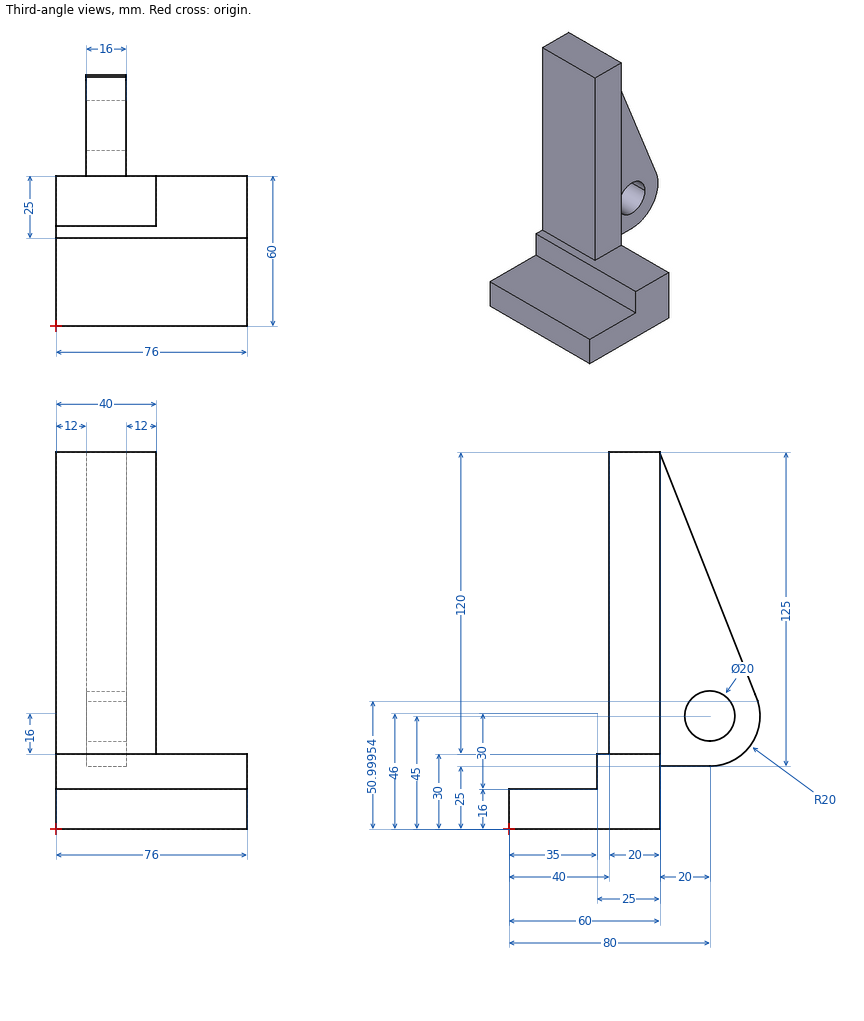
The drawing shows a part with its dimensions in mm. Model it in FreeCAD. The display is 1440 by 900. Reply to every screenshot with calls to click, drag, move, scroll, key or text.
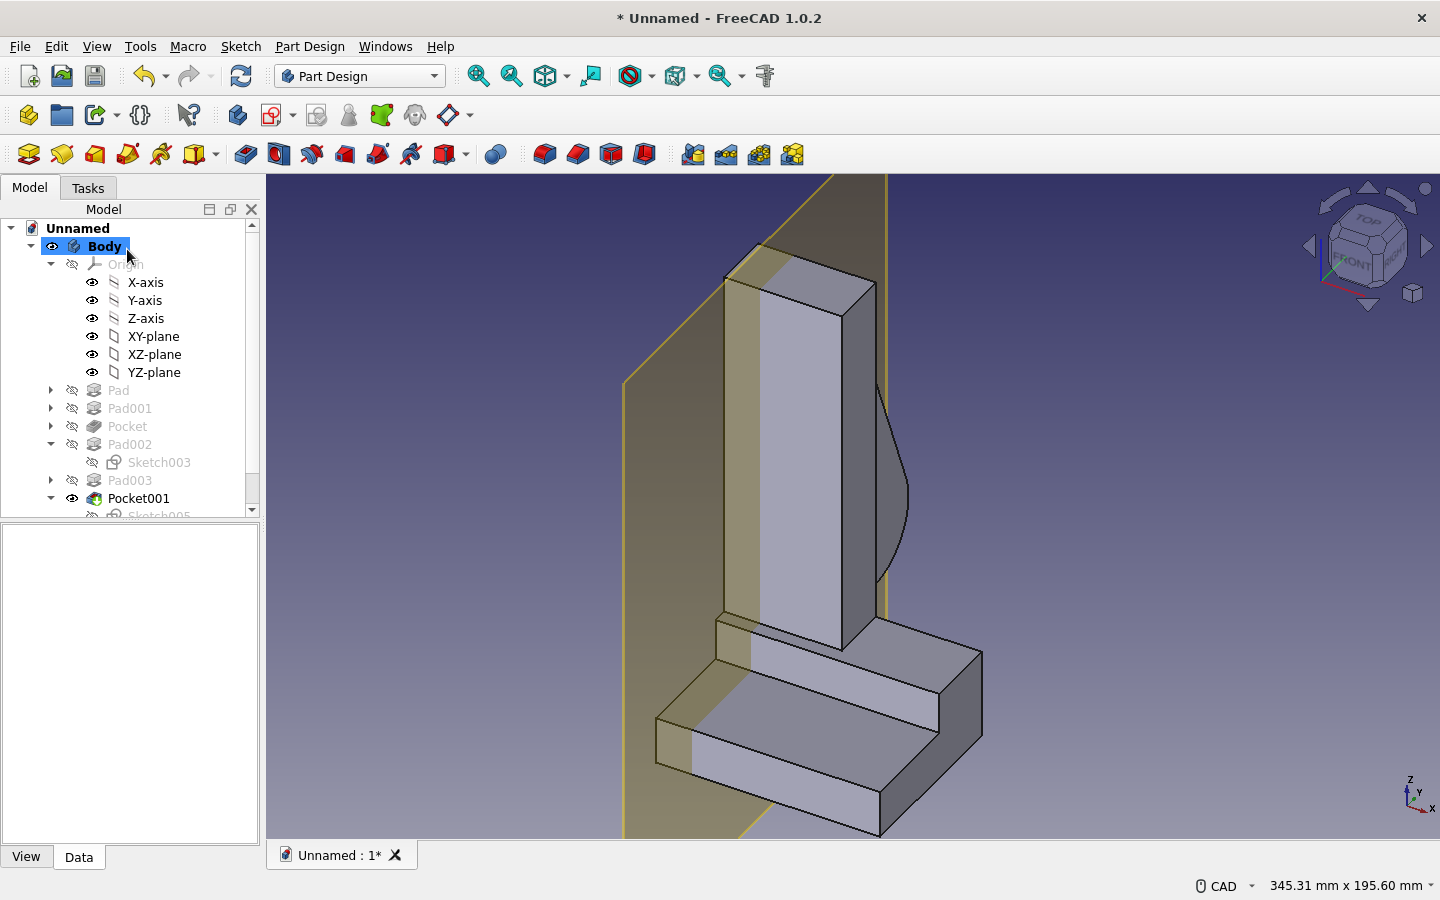
scroll(101, 368, down, 3)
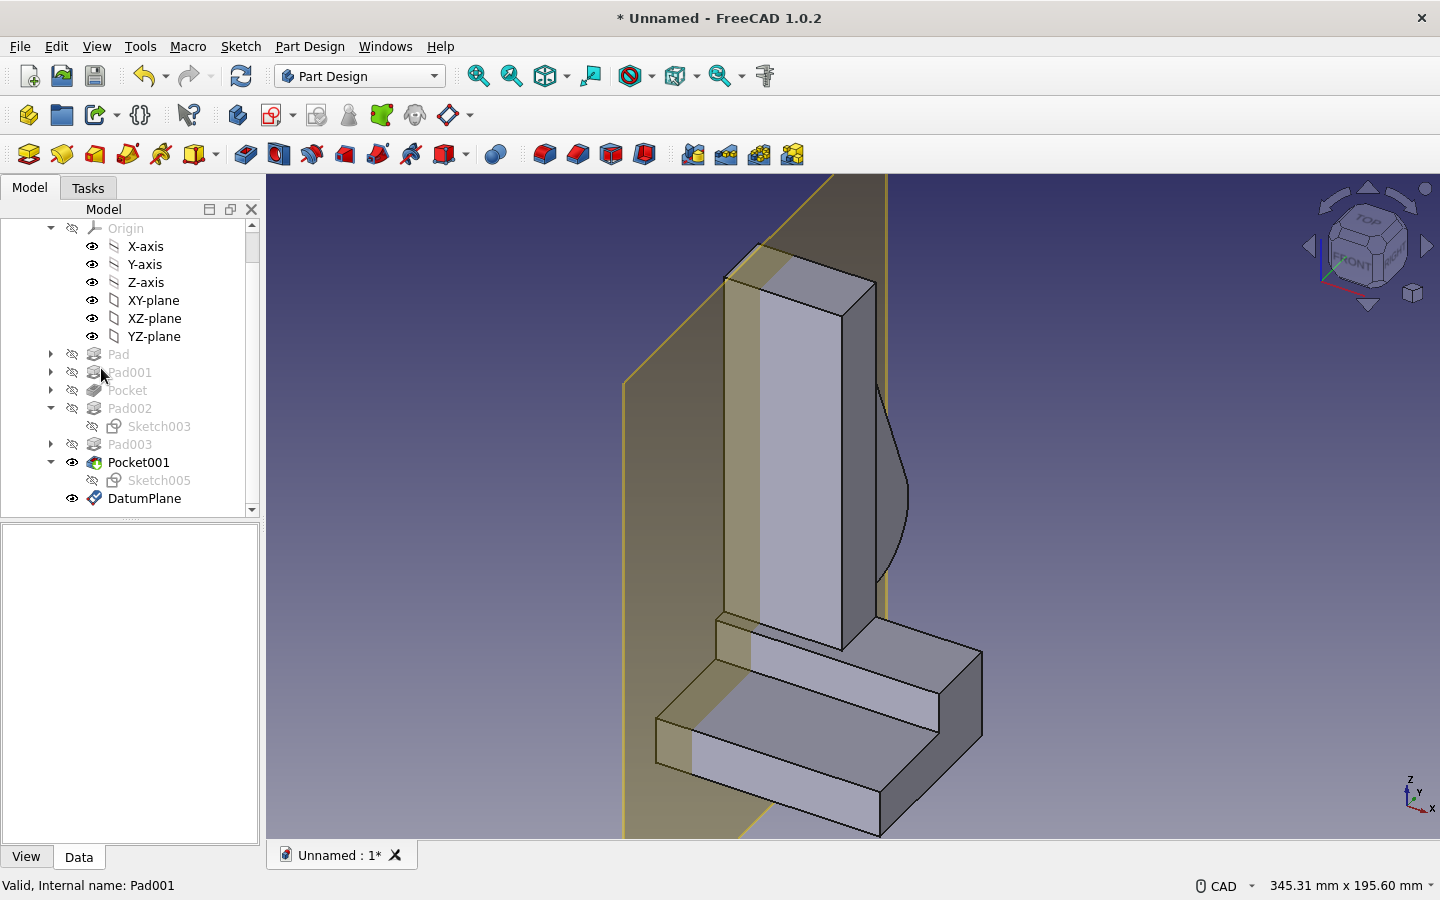
click(117, 498)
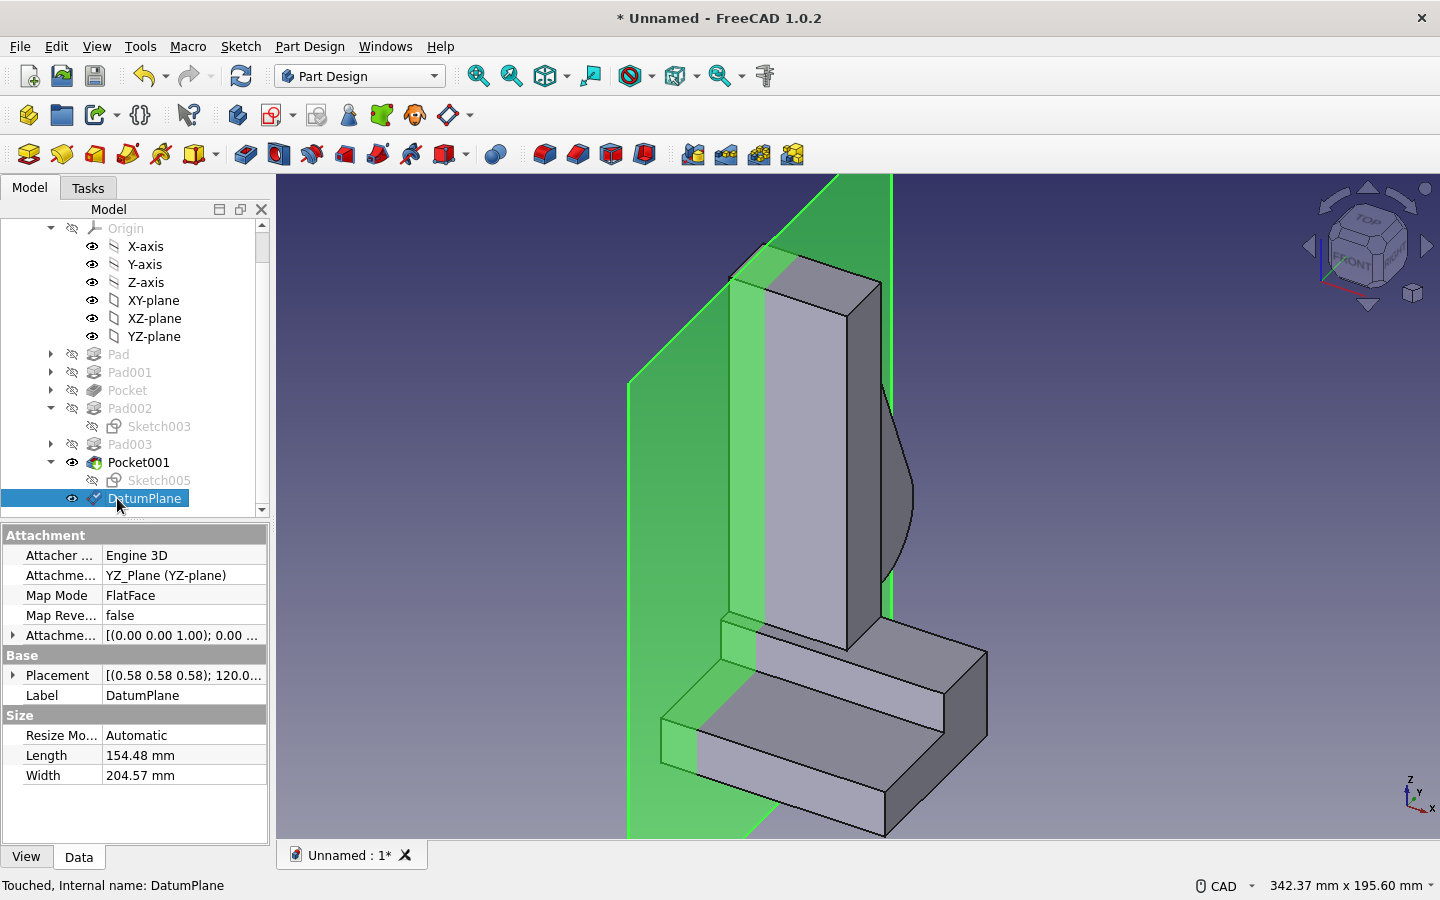
click(270, 116)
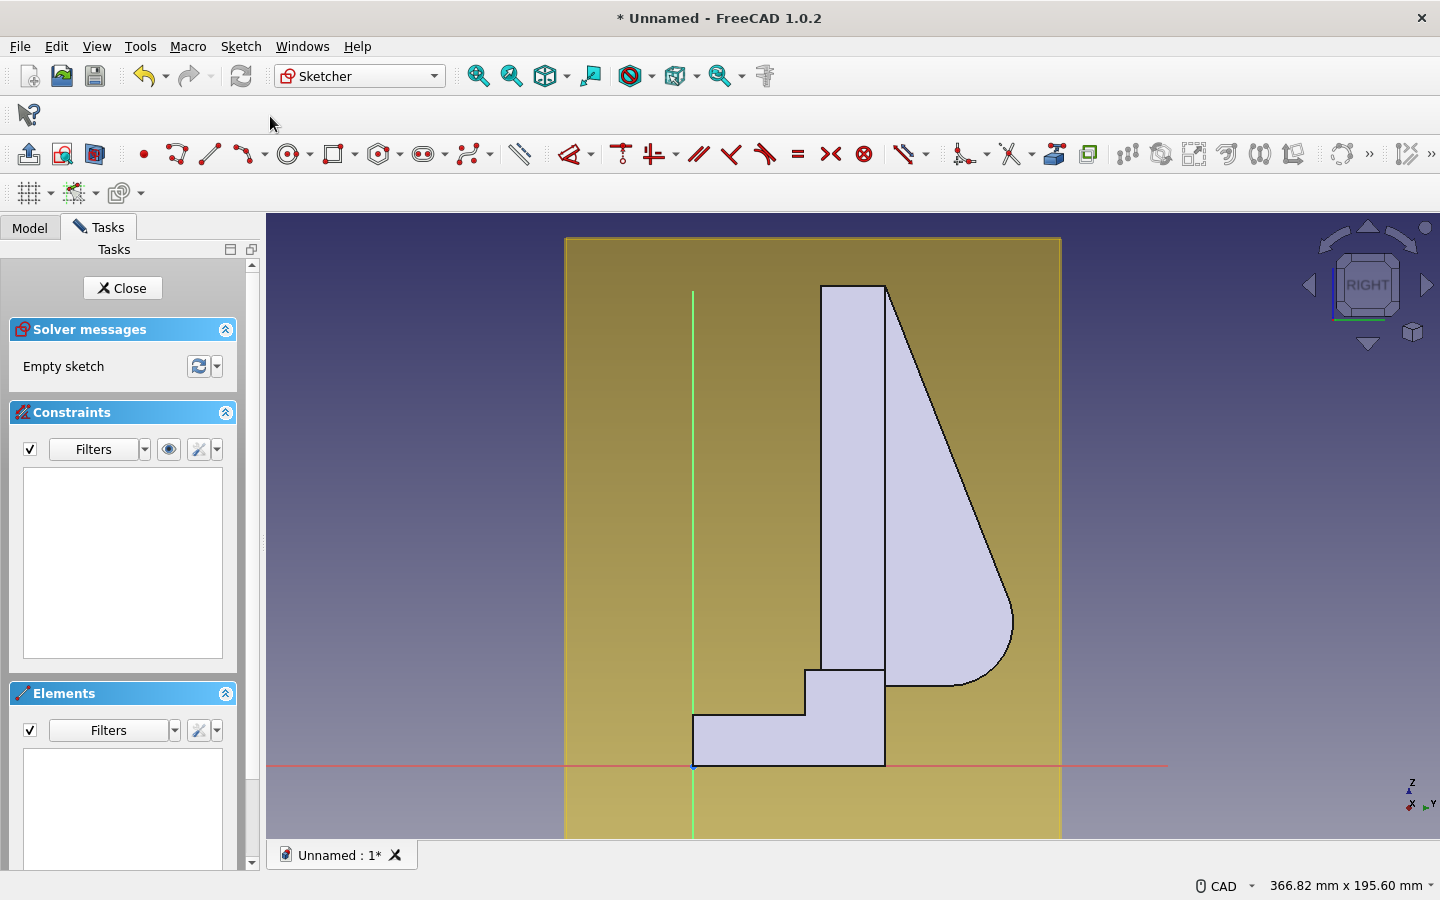
key(q)
key(s)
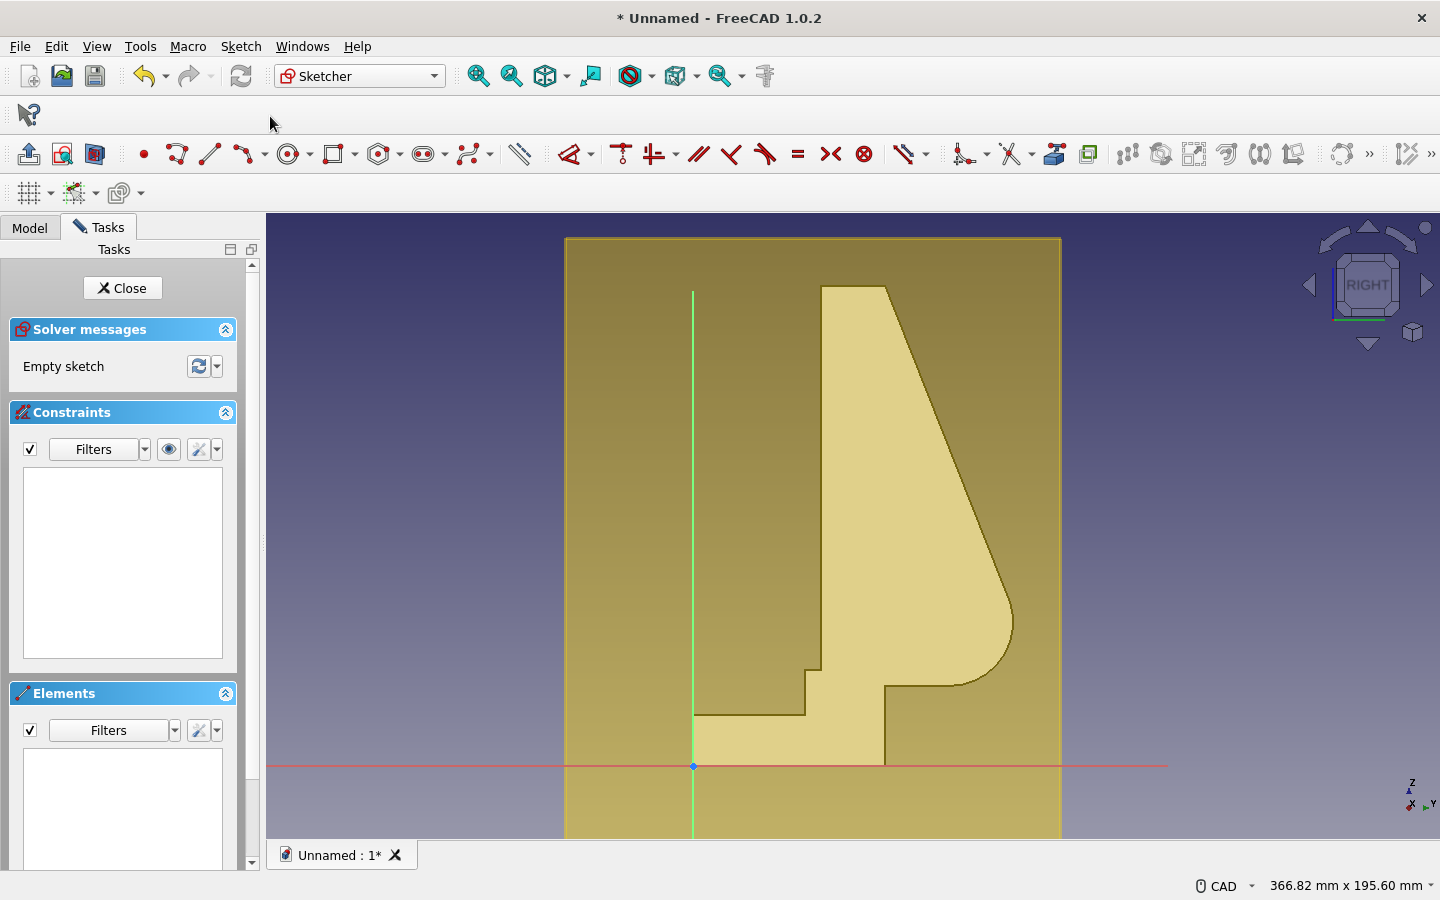
click(177, 154)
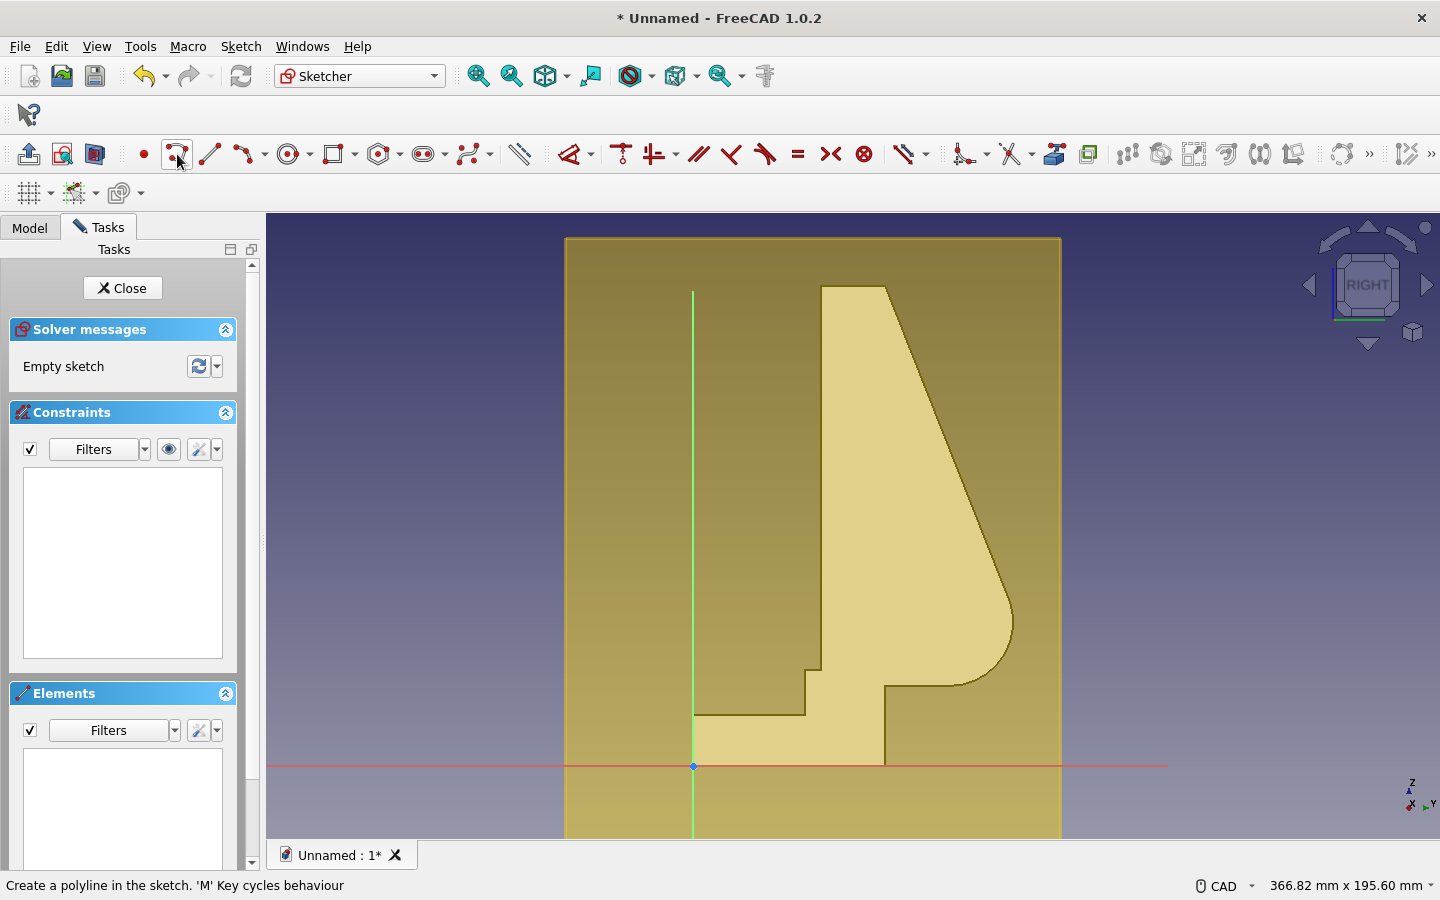
click(949, 686)
click(885, 686)
click(885, 286)
click(1010, 603)
right_click(1010, 603)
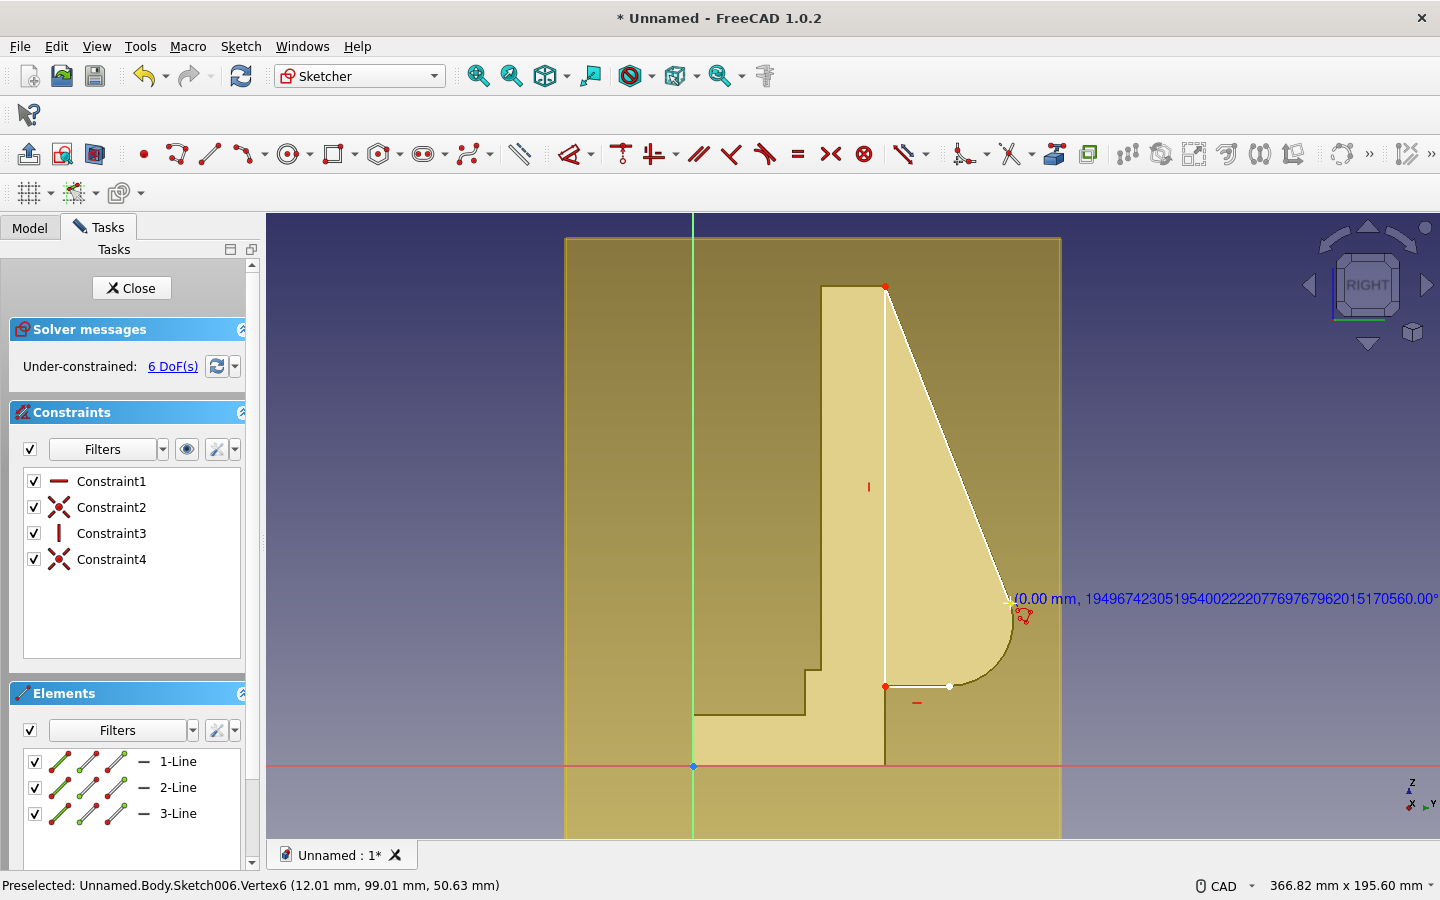
click(242, 154)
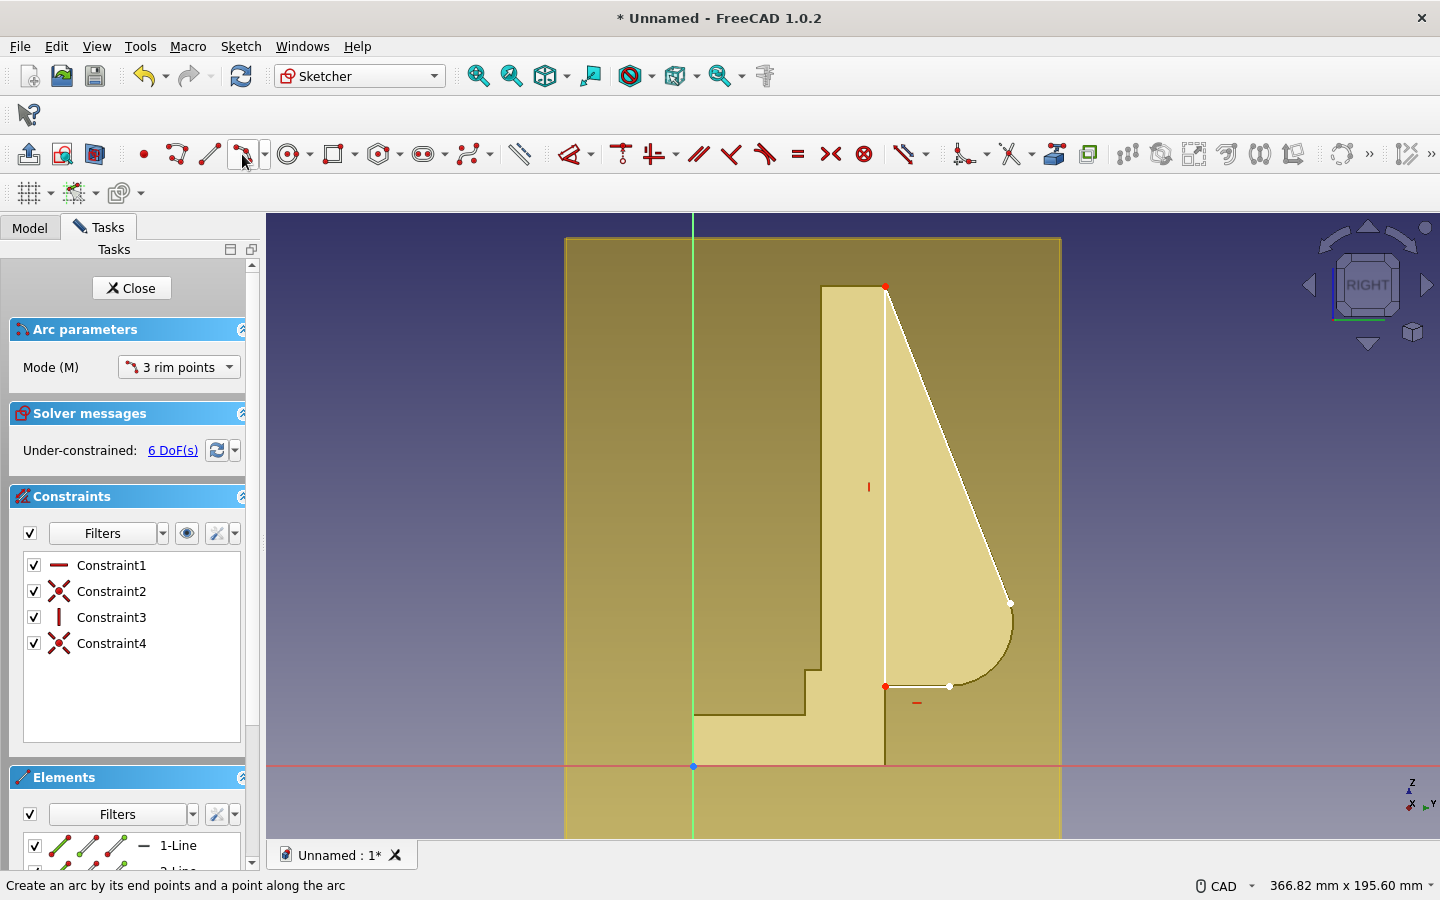
click(1010, 604)
click(949, 687)
click(1001, 660)
key(Escape)